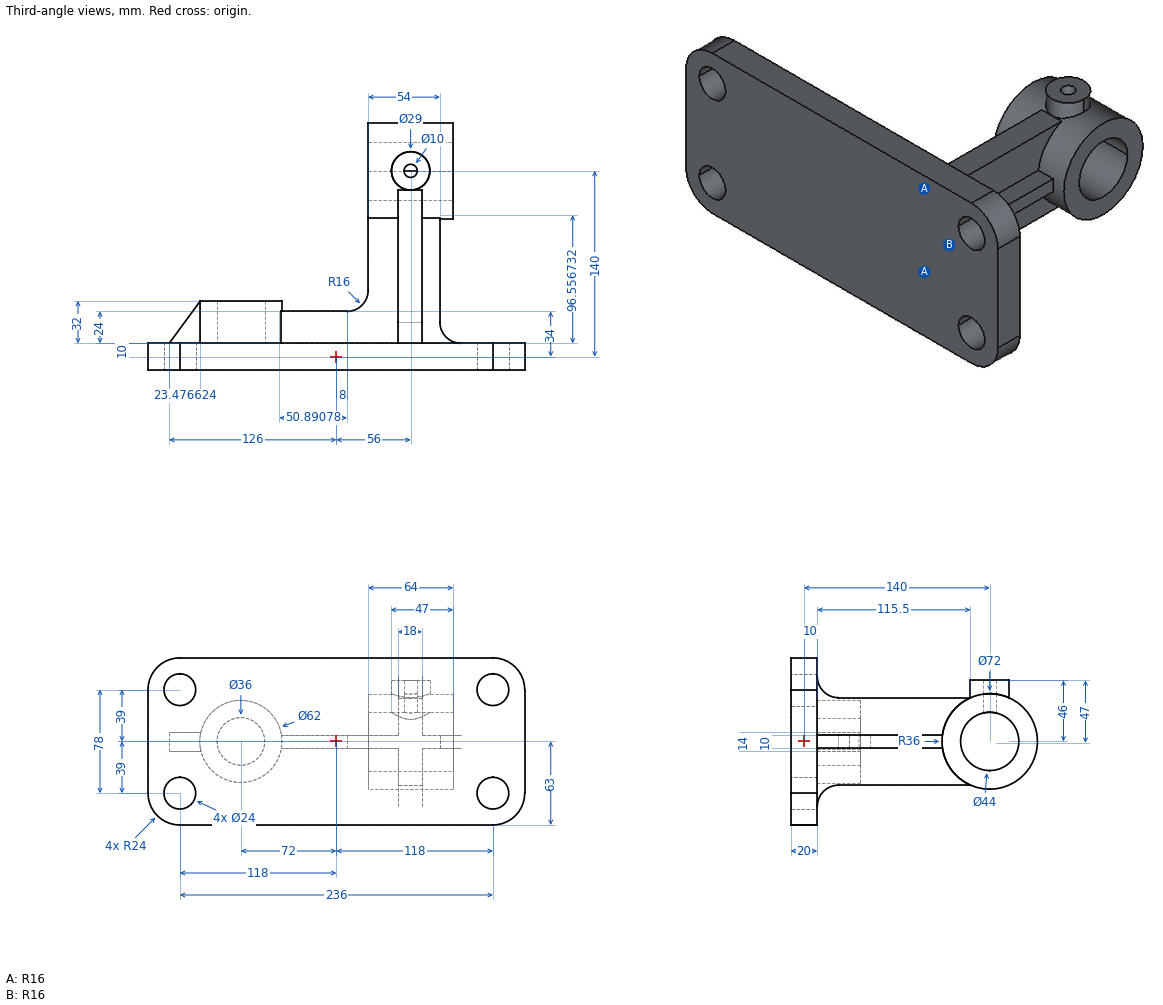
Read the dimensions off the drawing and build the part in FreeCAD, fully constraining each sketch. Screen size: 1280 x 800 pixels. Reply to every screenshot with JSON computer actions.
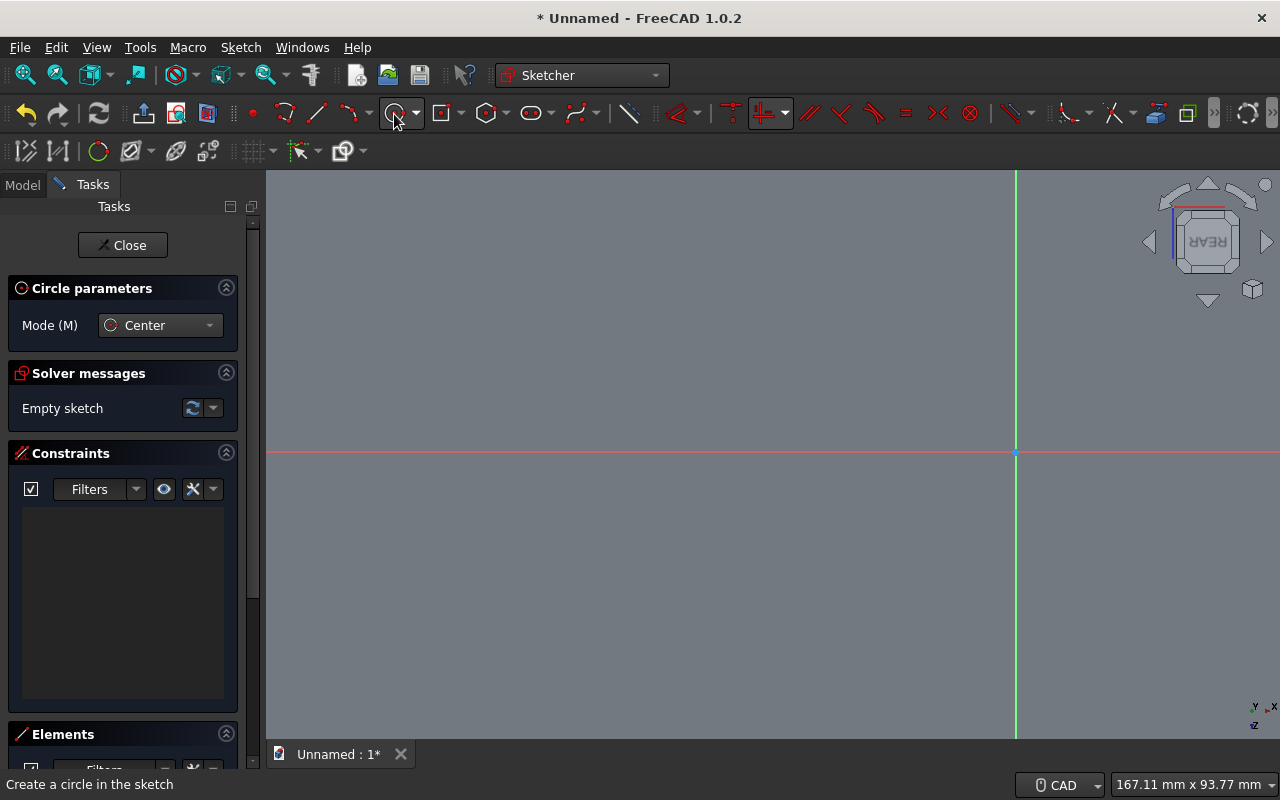
{"action": "left_click", "coordinate": [579, 452]}
{"action": "mouse_move", "coordinate": [712, 319]}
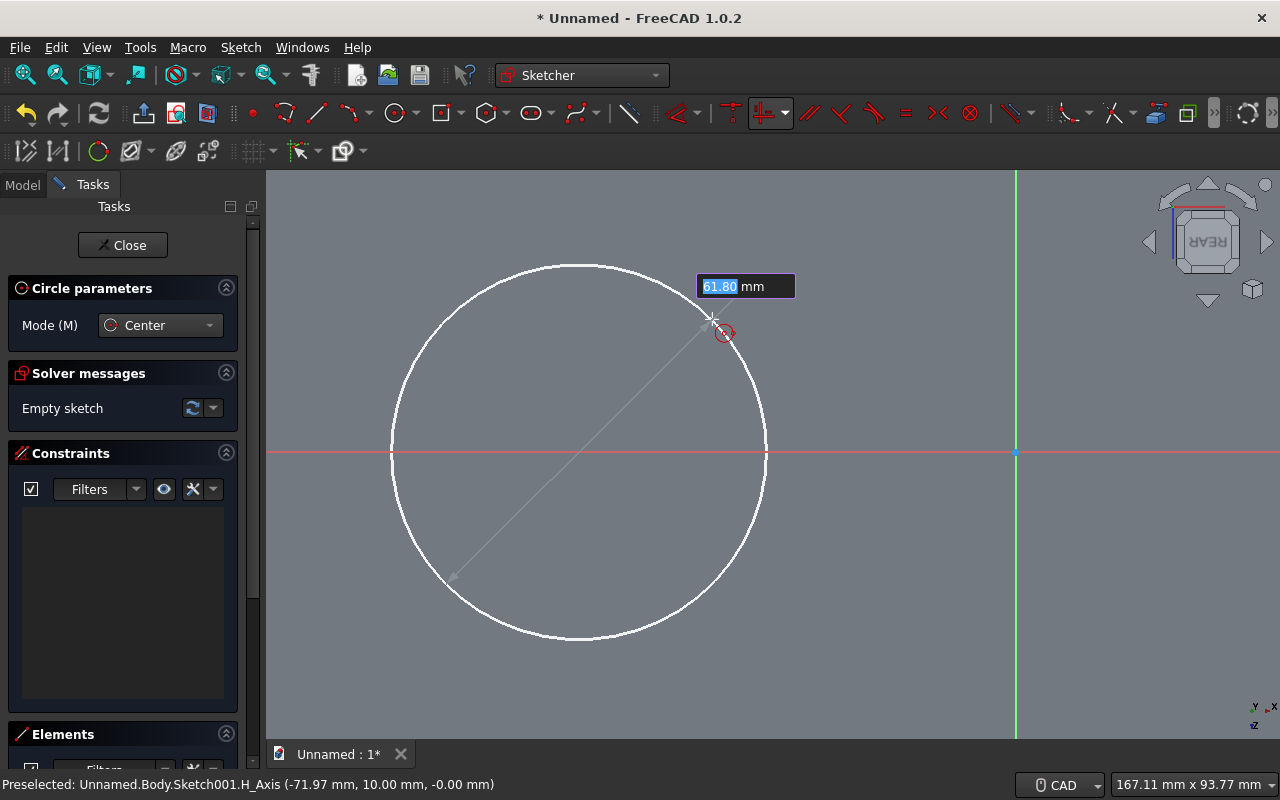
{"action": "type", "text": "62"}
{"action": "key", "text": "Return"}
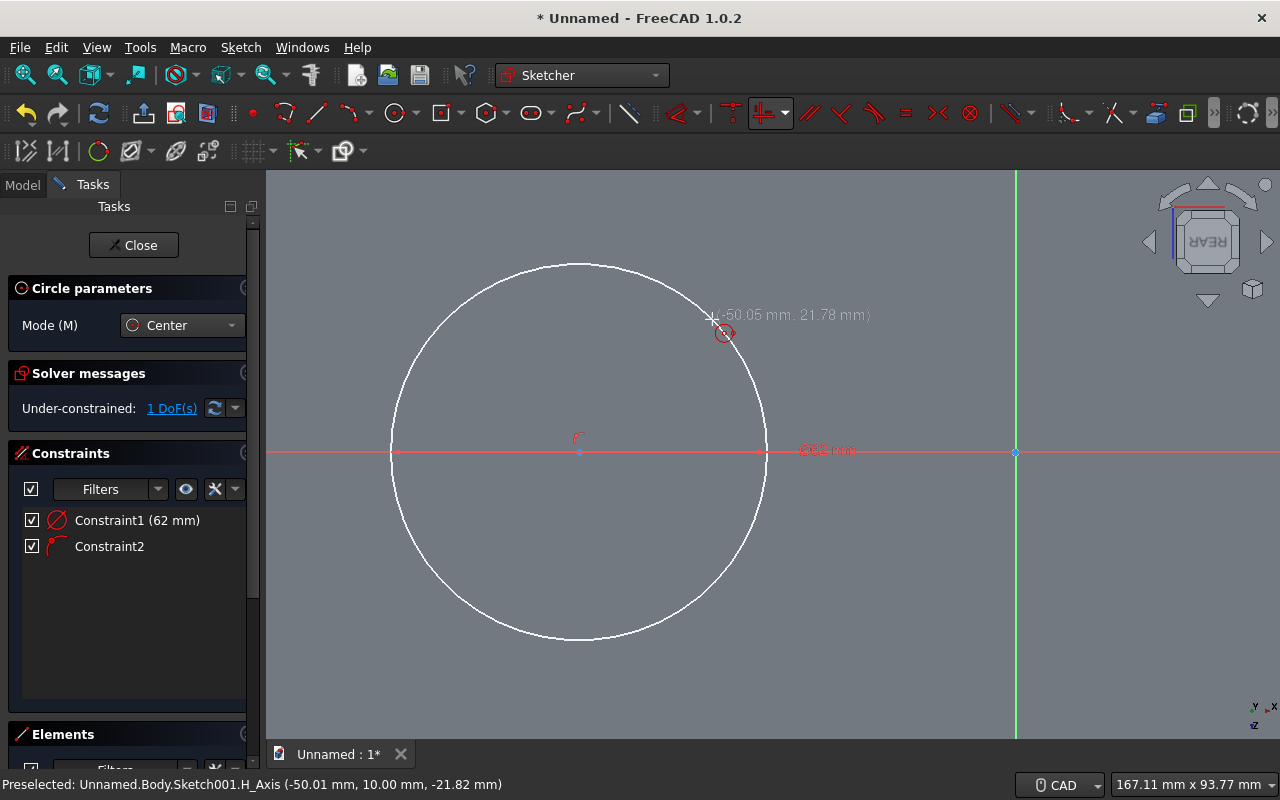
{"action": "left_click", "coordinate": [579, 452]}
{"action": "mouse_move", "coordinate": [656, 375]}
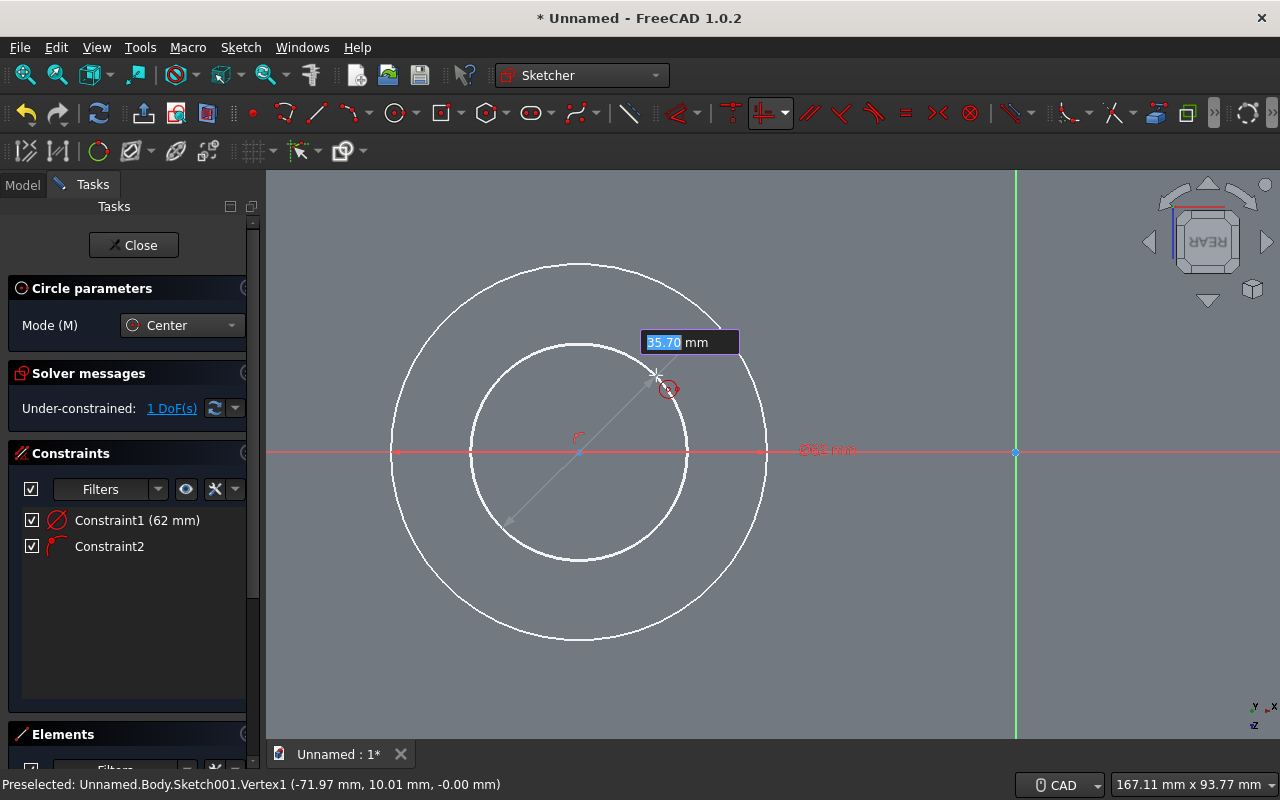
{"action": "type", "text": "36"}
{"action": "key", "text": "Return"}
{"action": "key", "text": "Escape"}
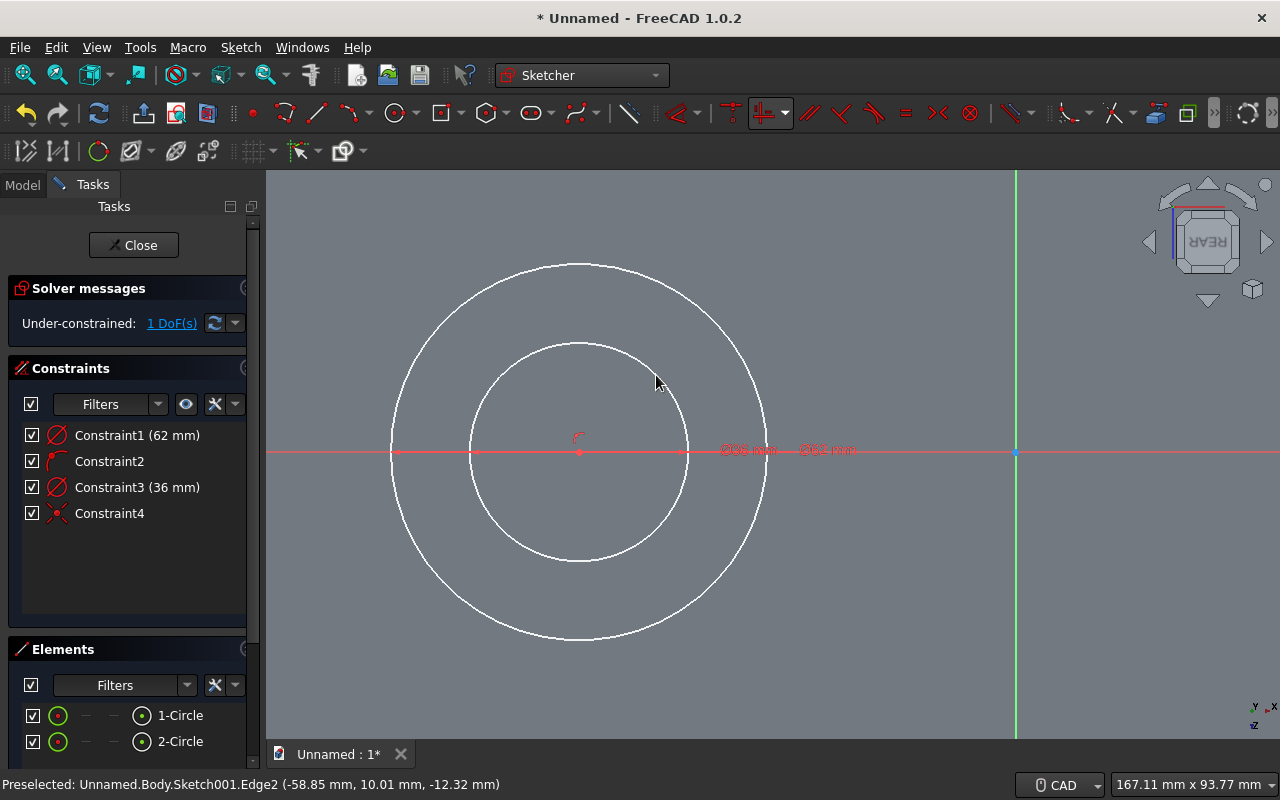
{"action": "left_click", "coordinate": [676, 114]}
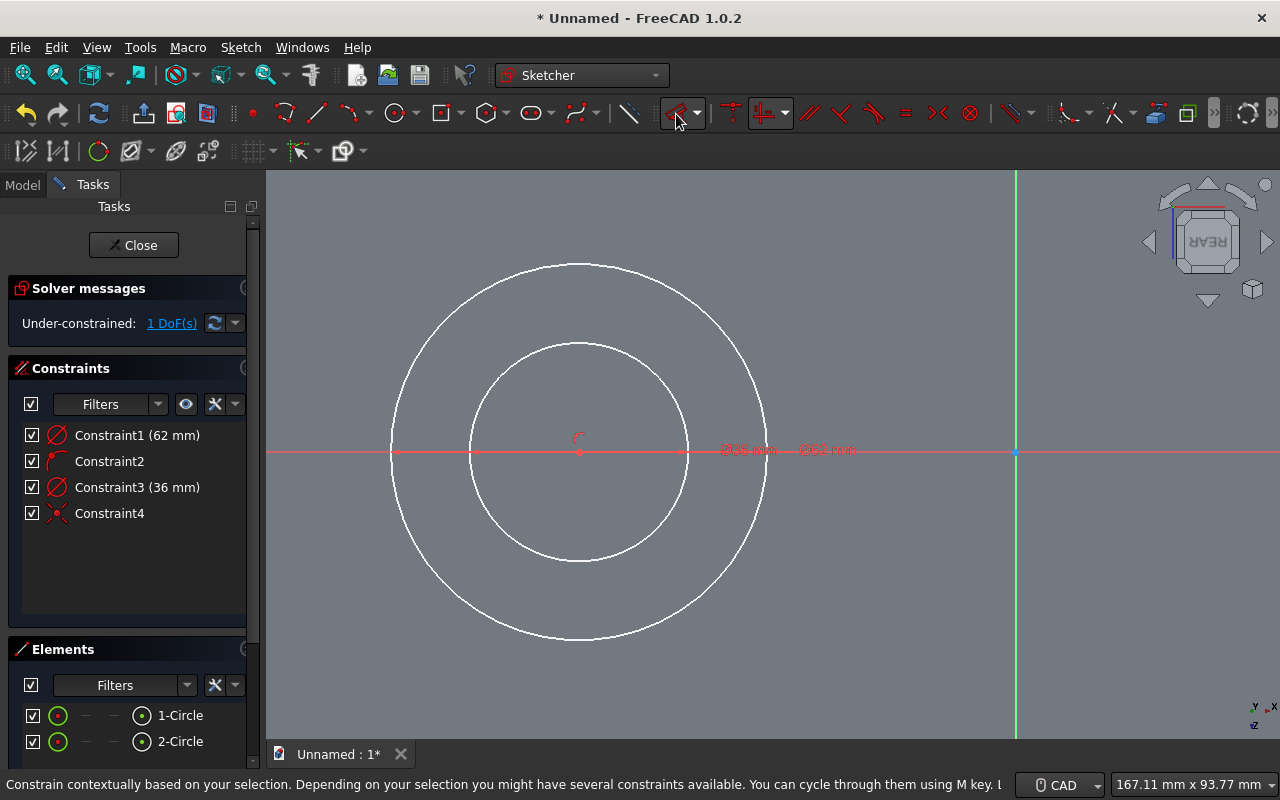
{"action": "left_click", "coordinate": [579, 452]}
{"action": "left_click", "coordinate": [797, 486]}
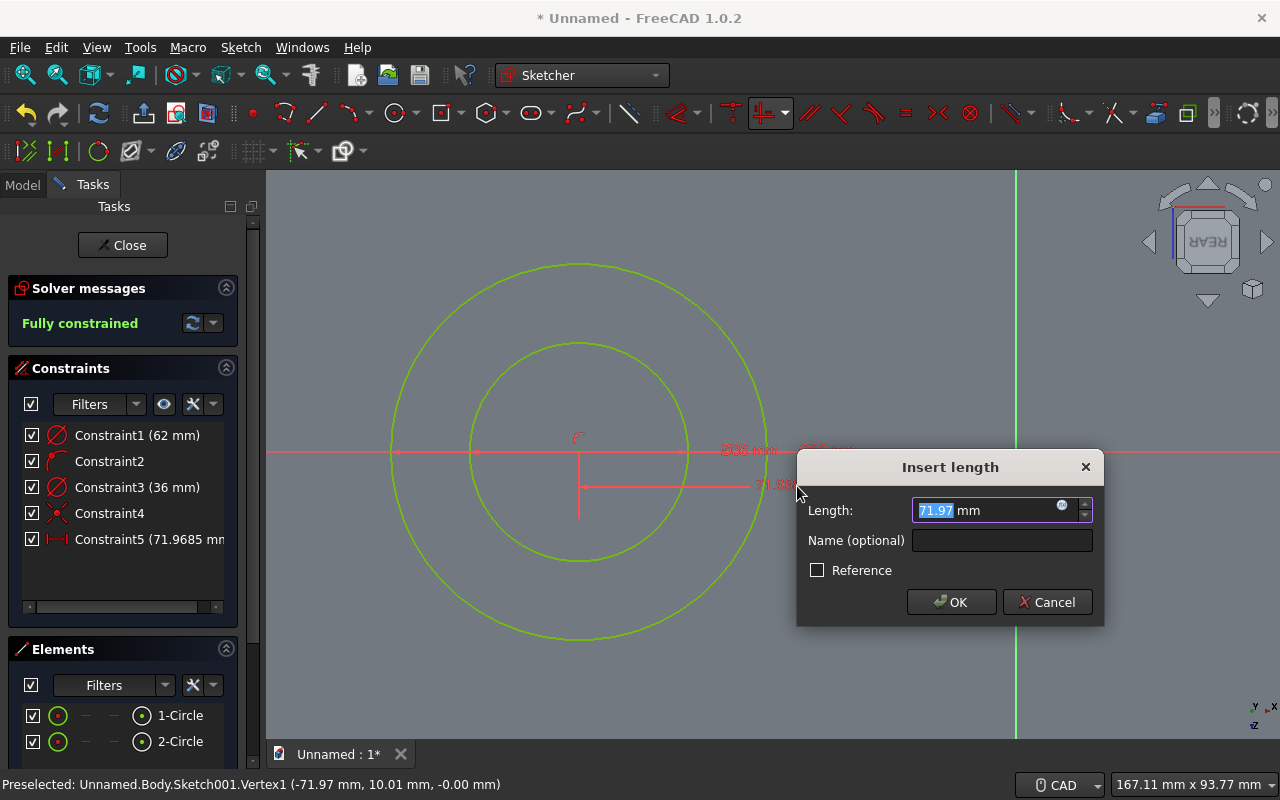
{"action": "type", "text": "72"}
{"action": "key", "text": "Return"}
{"action": "key", "text": "Escape"}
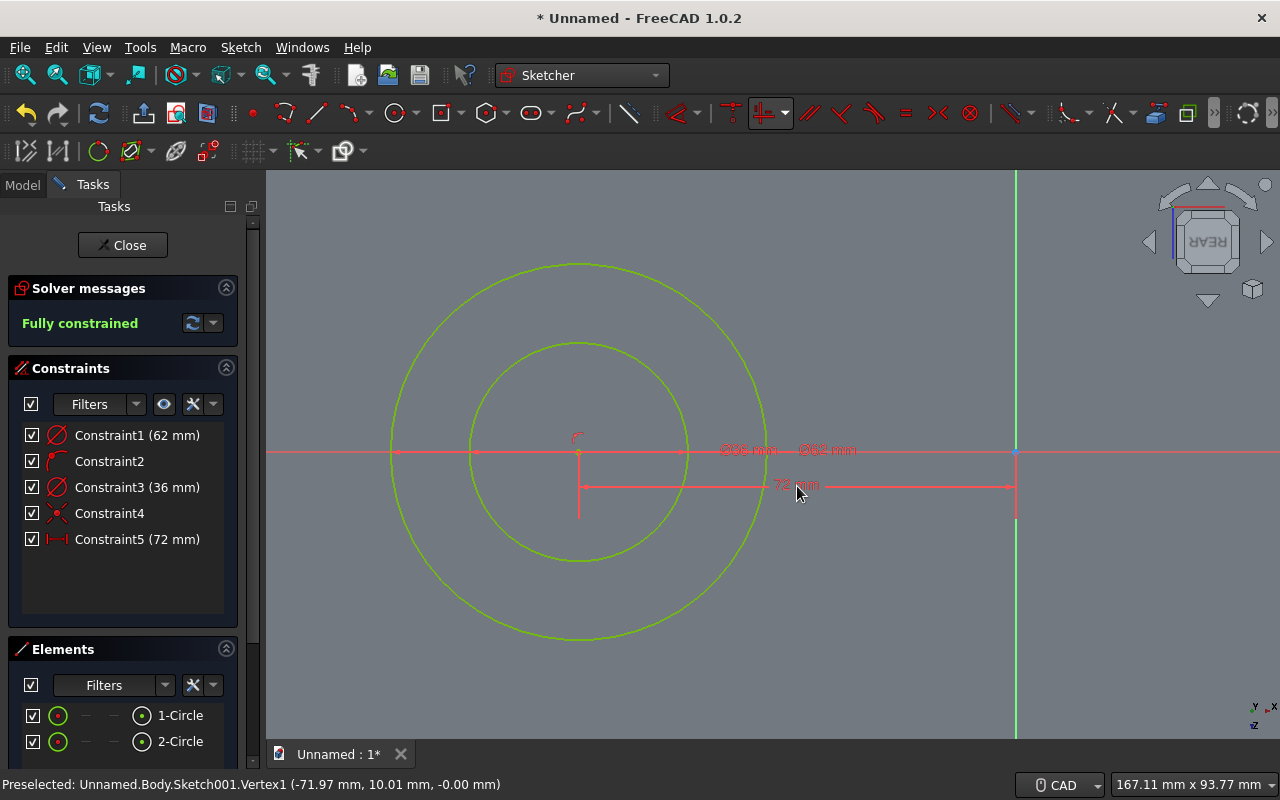
{"action": "left_click", "coordinate": [123, 245]}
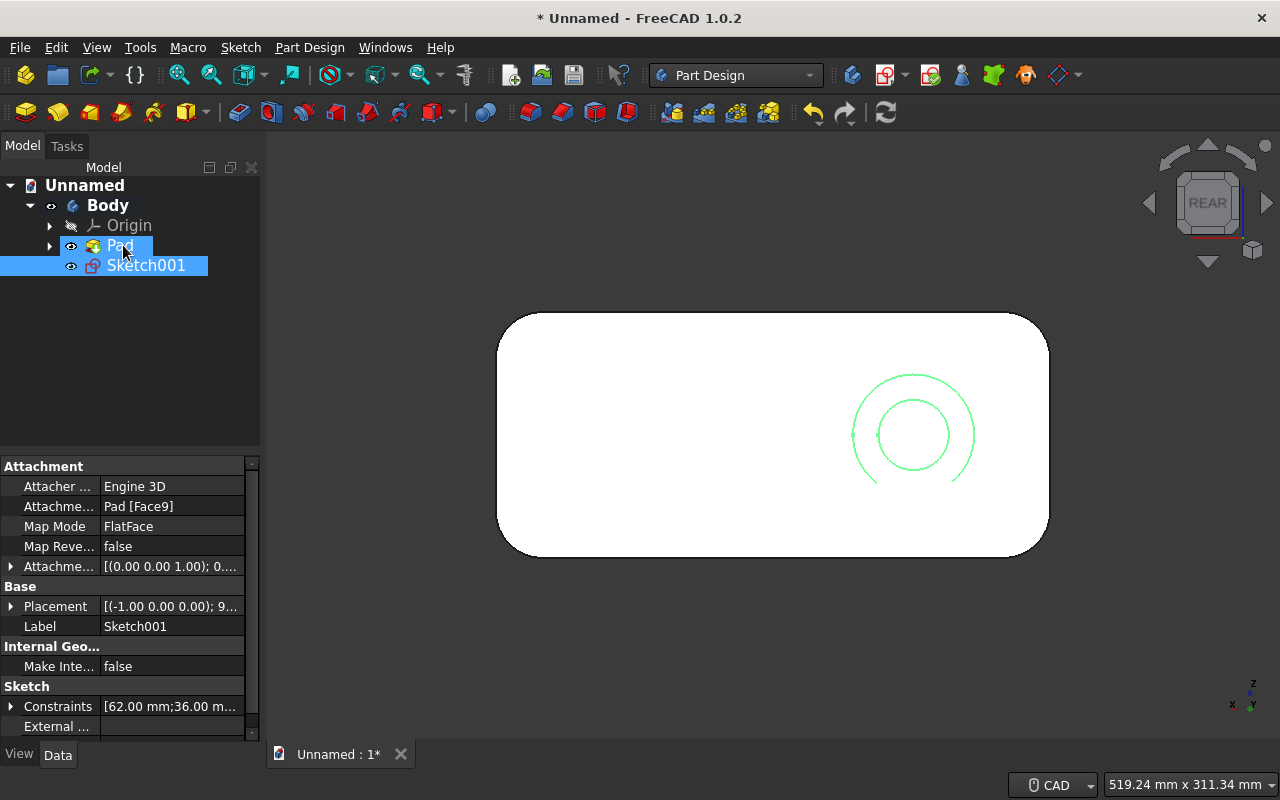
{"action": "left_click", "coordinate": [26, 112]}